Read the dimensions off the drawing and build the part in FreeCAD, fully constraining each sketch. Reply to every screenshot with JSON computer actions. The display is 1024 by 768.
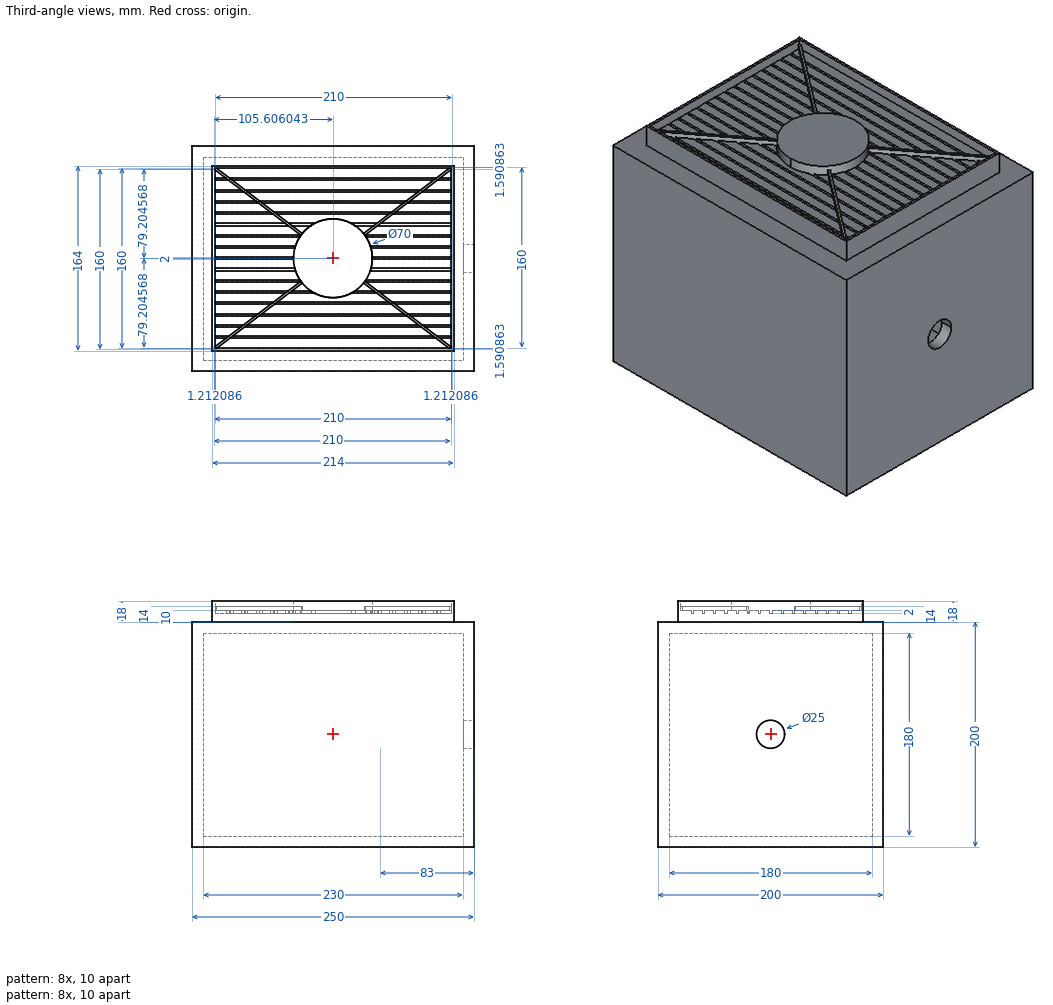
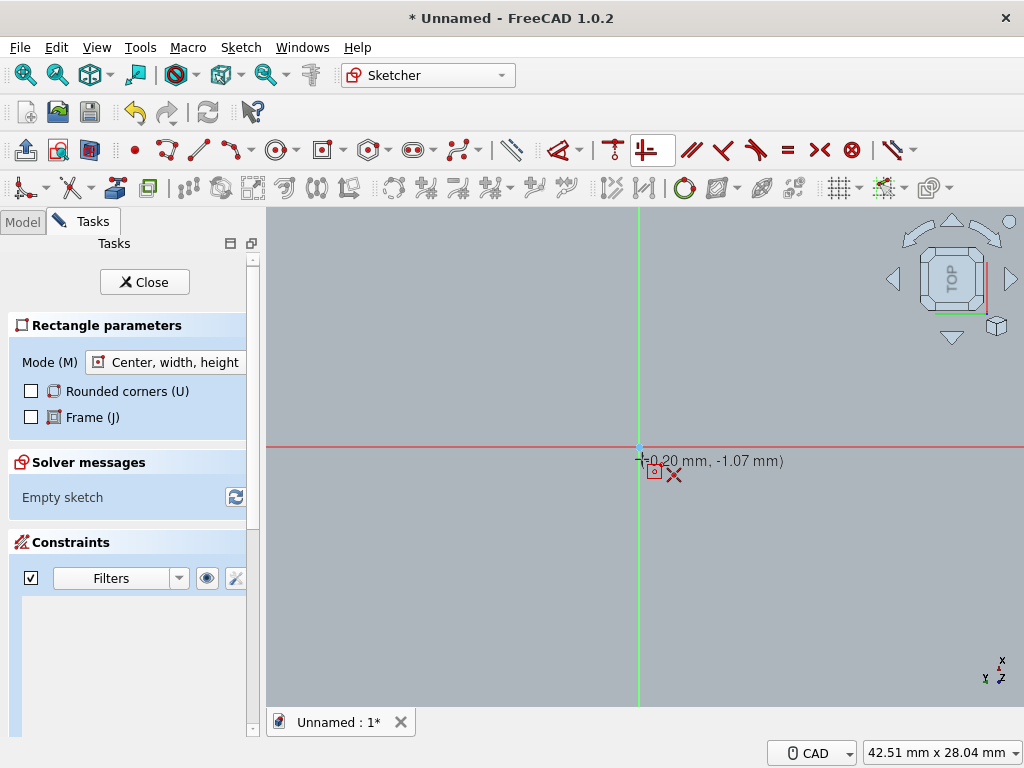
{"action": "scroll", "coordinate": [570, 458], "scroll_direction": "down", "scroll_amount": 12}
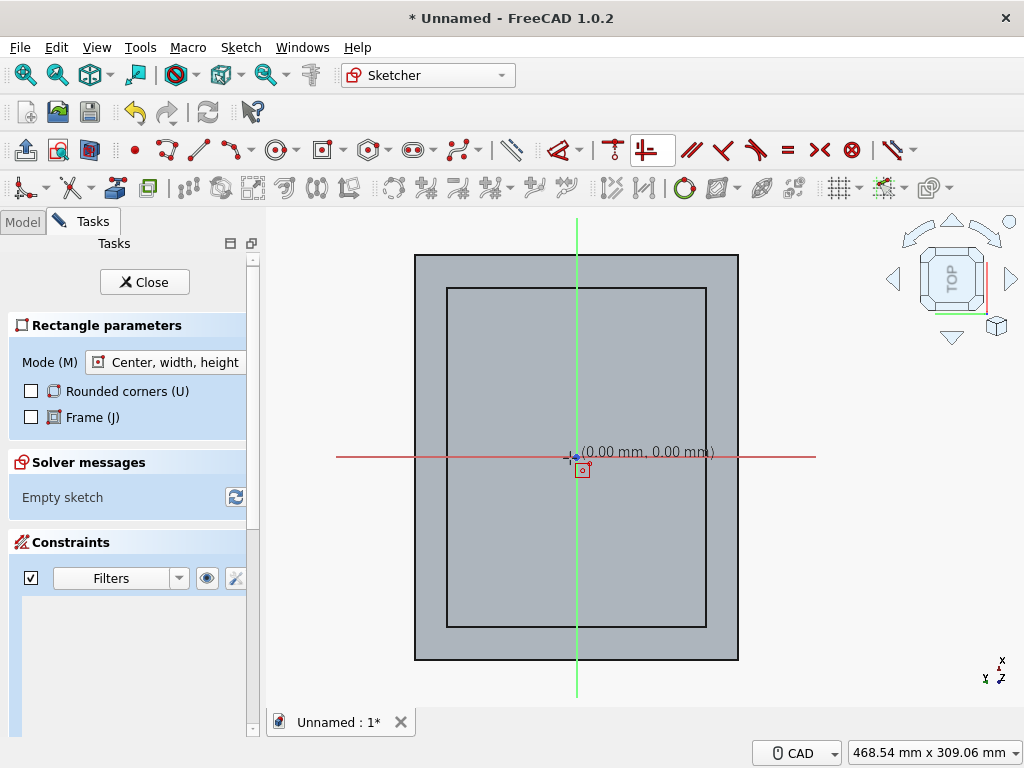
{"action": "left_click", "coordinate": [577, 457]}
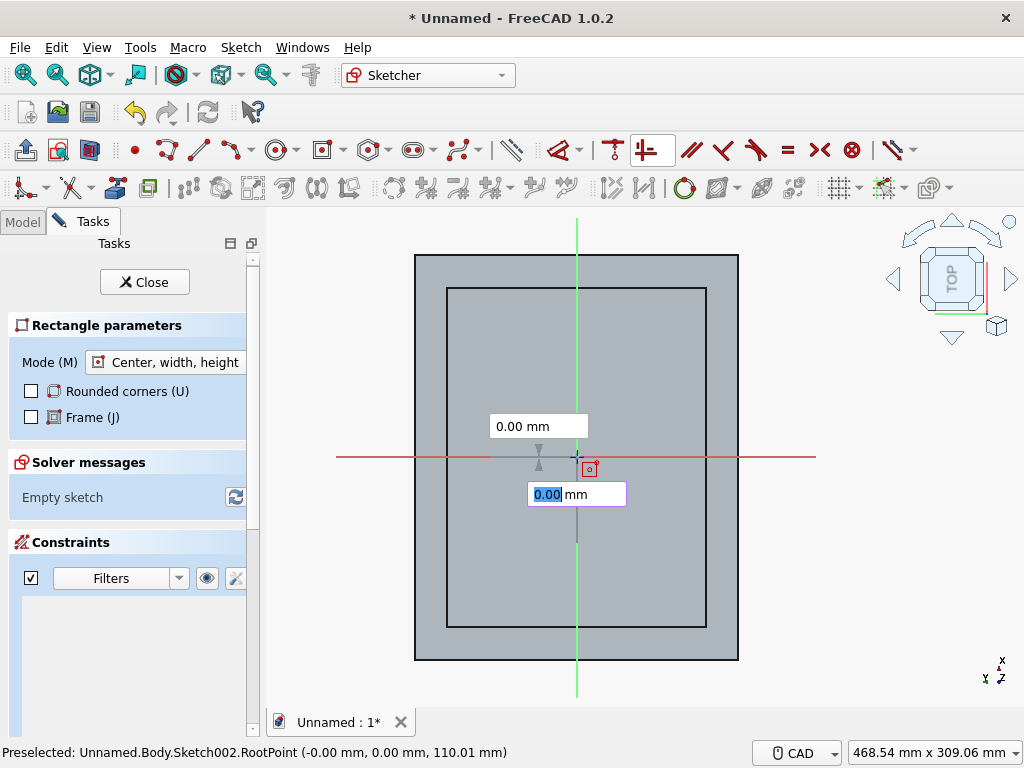
{"action": "scroll", "coordinate": [578, 288], "scroll_direction": "up", "scroll_amount": 12}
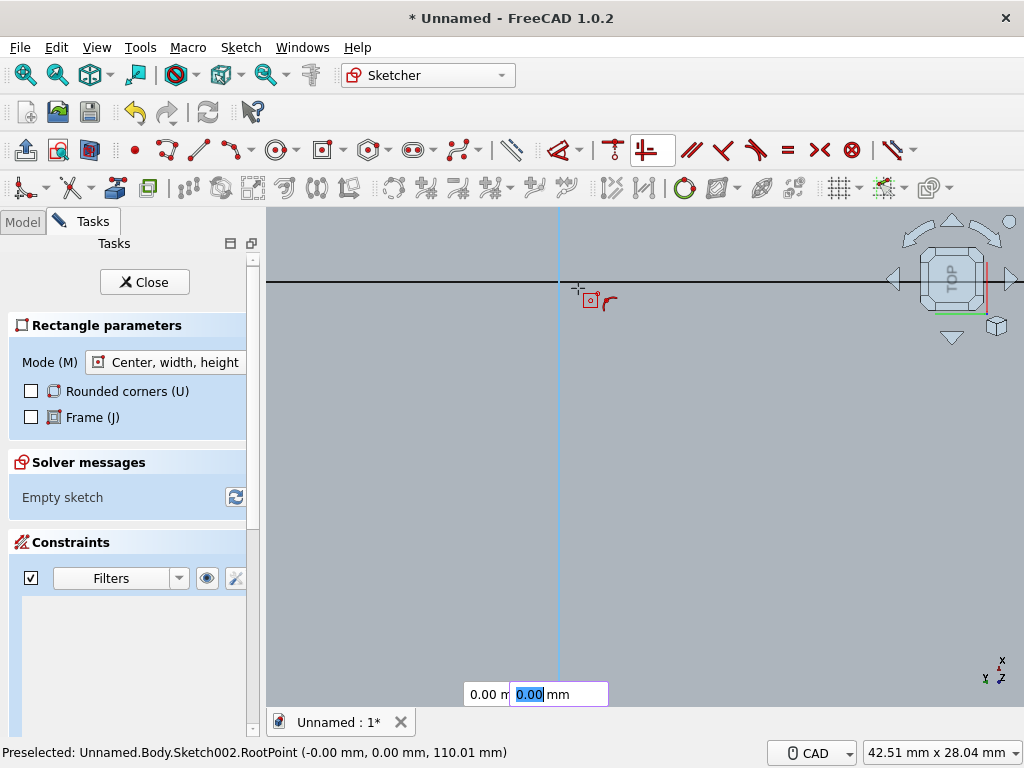
{"action": "left_click", "coordinate": [577, 282]}
{"action": "key", "text": "Escape"}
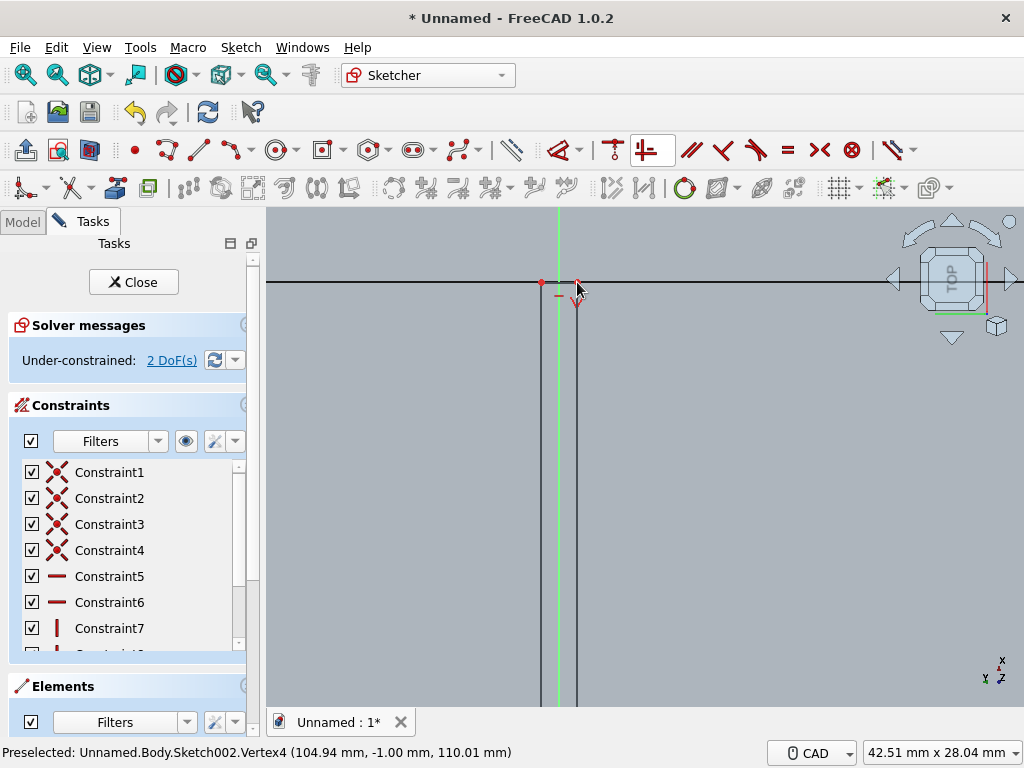
{"action": "left_click", "coordinate": [558, 150]}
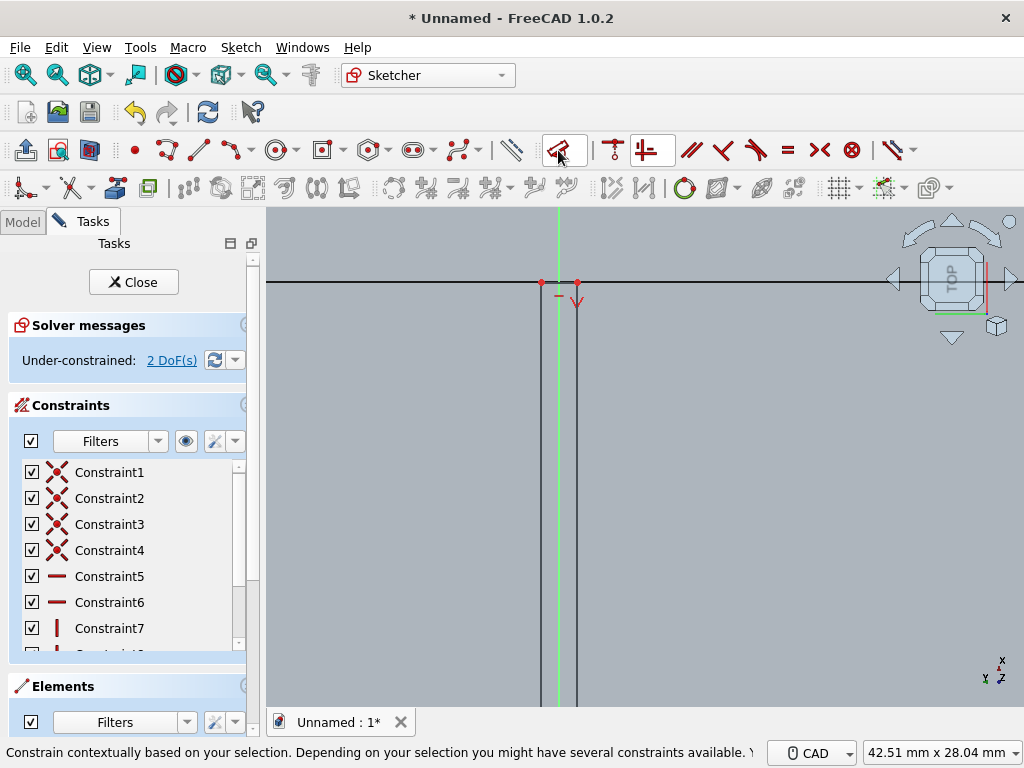
{"action": "scroll", "coordinate": [578, 288], "scroll_direction": "down", "scroll_amount": 12}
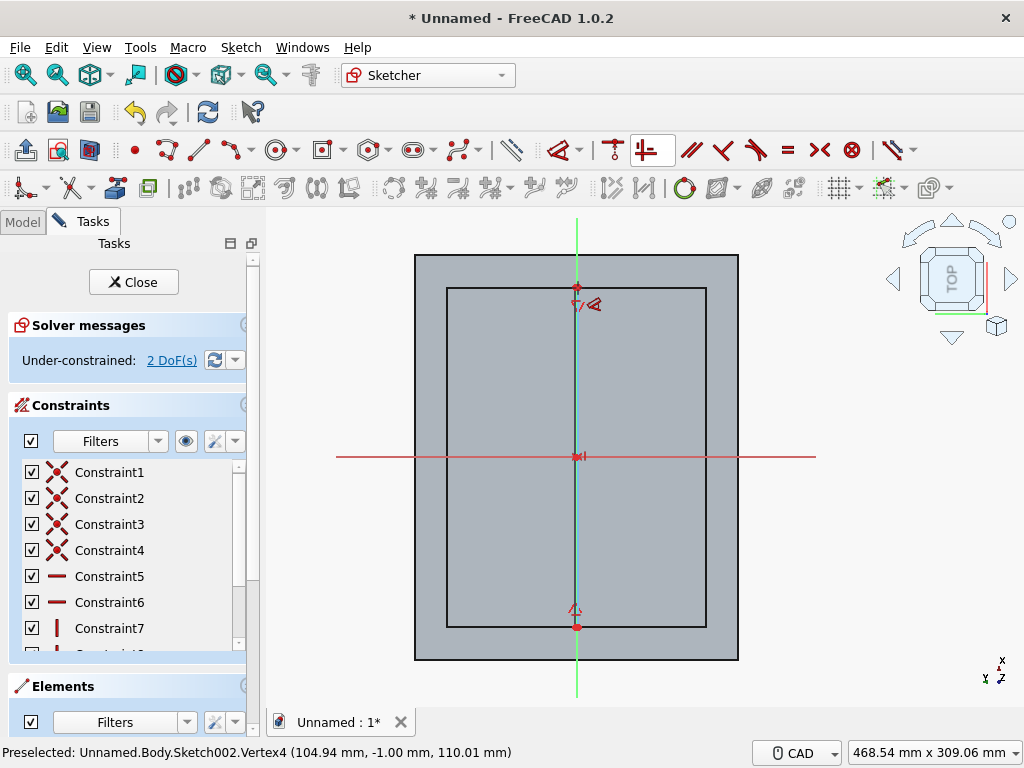
{"action": "scroll", "coordinate": [576, 627], "scroll_direction": "up", "scroll_amount": 13}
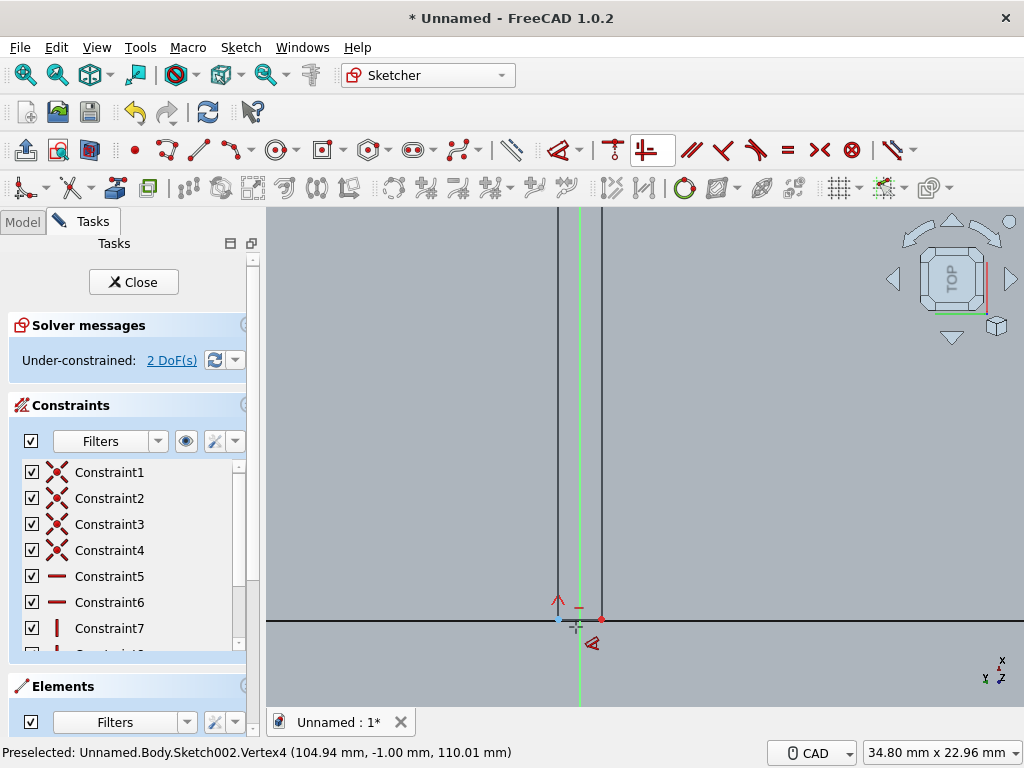
{"action": "left_click", "coordinate": [575, 620]}
{"action": "left_click", "coordinate": [565, 654]}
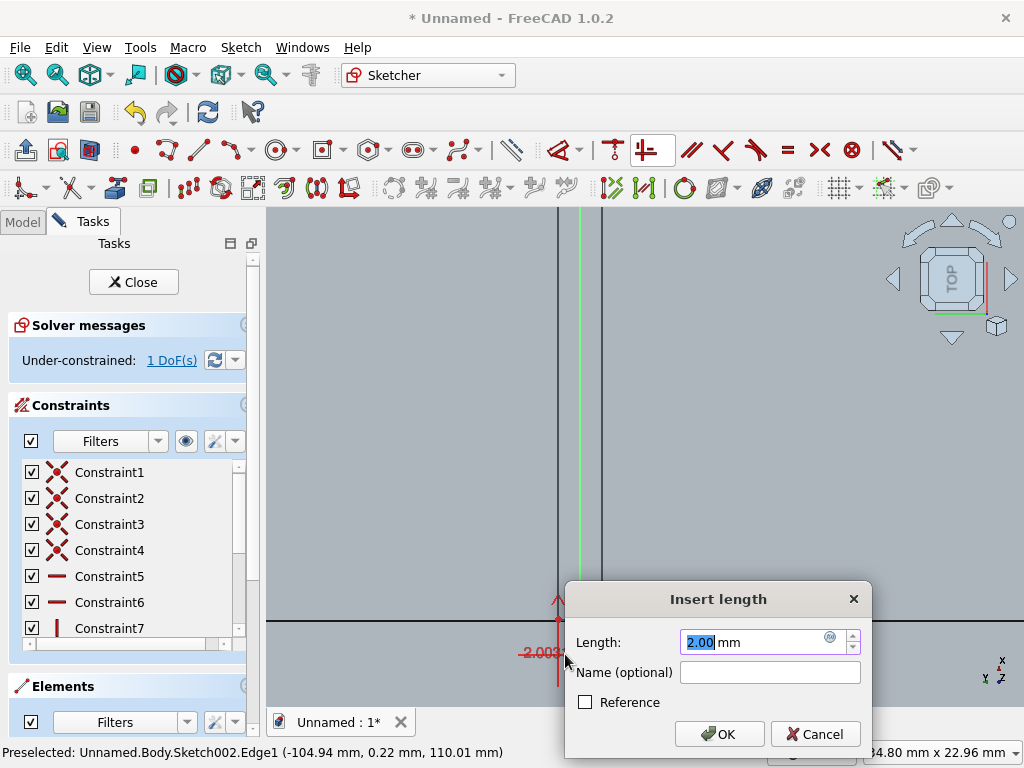
{"action": "type", "text": "2"}
{"action": "key", "text": "Return"}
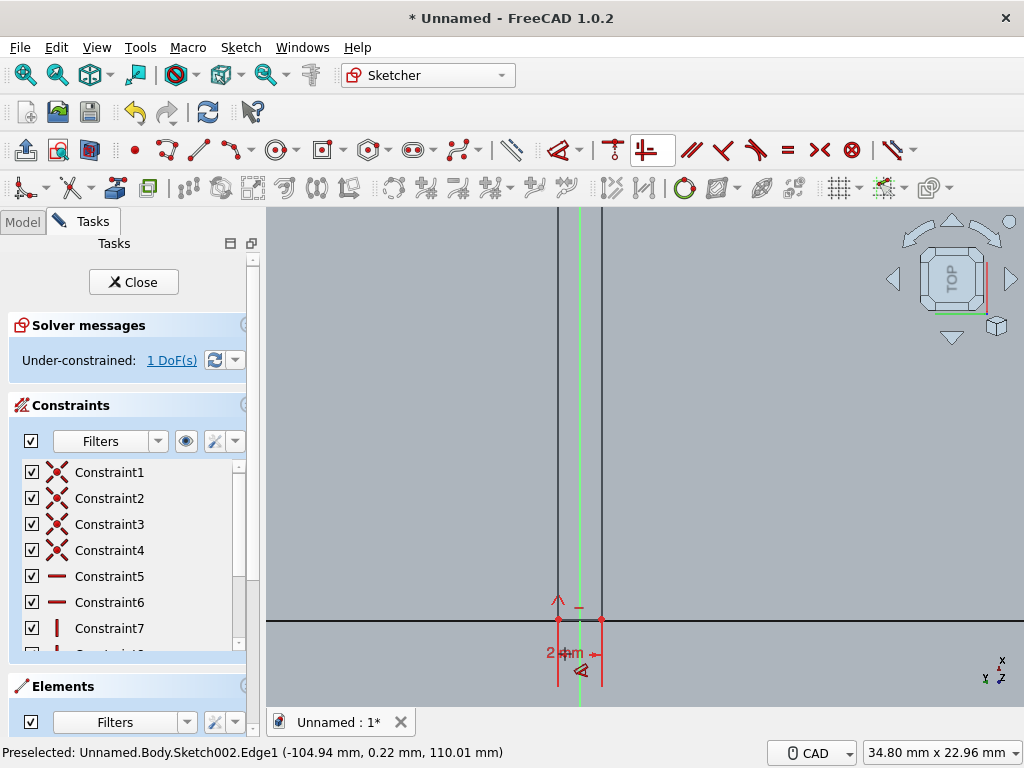
{"action": "scroll", "coordinate": [576, 627], "scroll_direction": "down", "scroll_amount": 13}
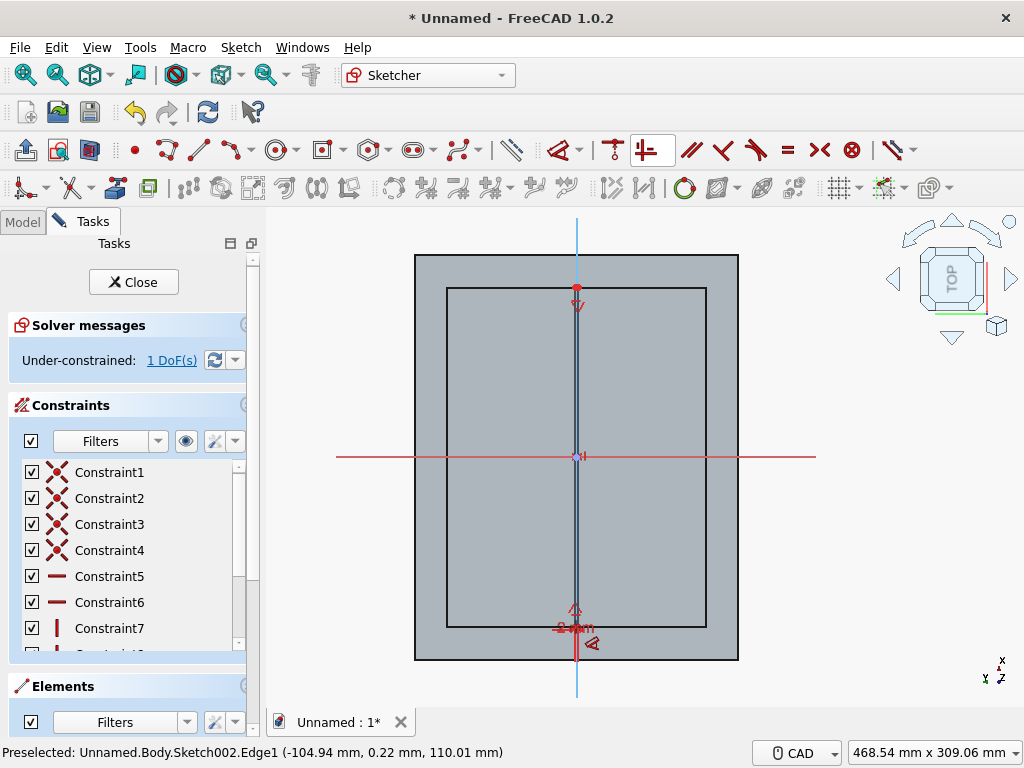
{"action": "scroll", "coordinate": [578, 525], "scroll_direction": "up", "scroll_amount": 11}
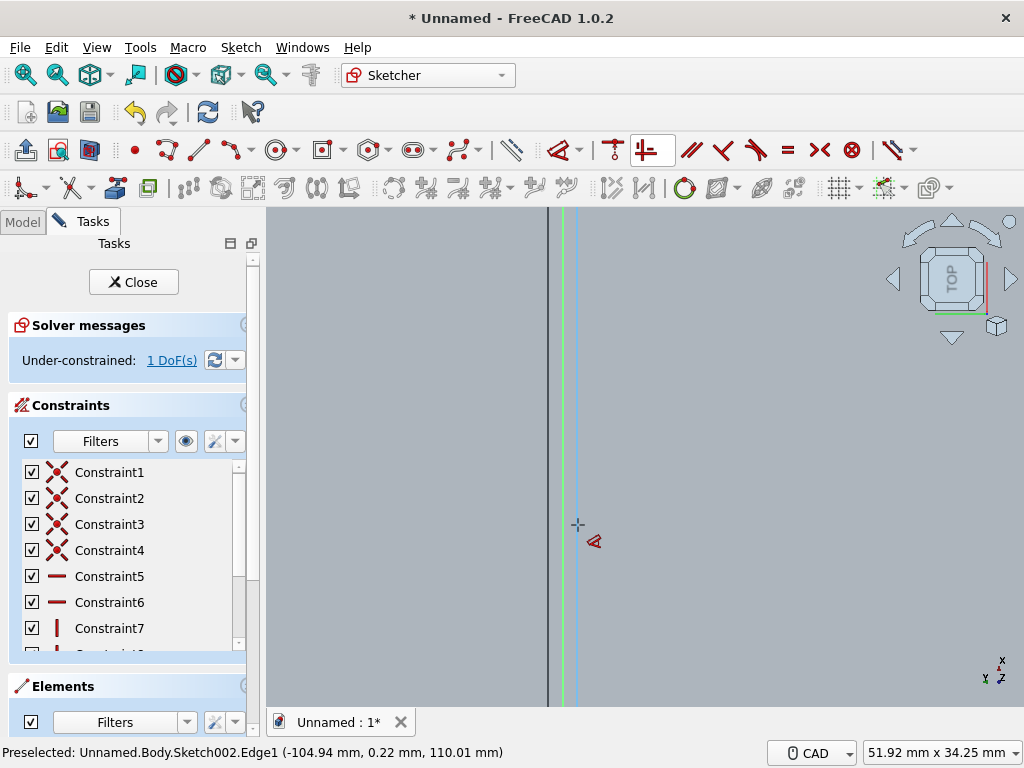
{"action": "left_click", "coordinate": [577, 523]}
{"action": "left_click", "coordinate": [611, 457]}